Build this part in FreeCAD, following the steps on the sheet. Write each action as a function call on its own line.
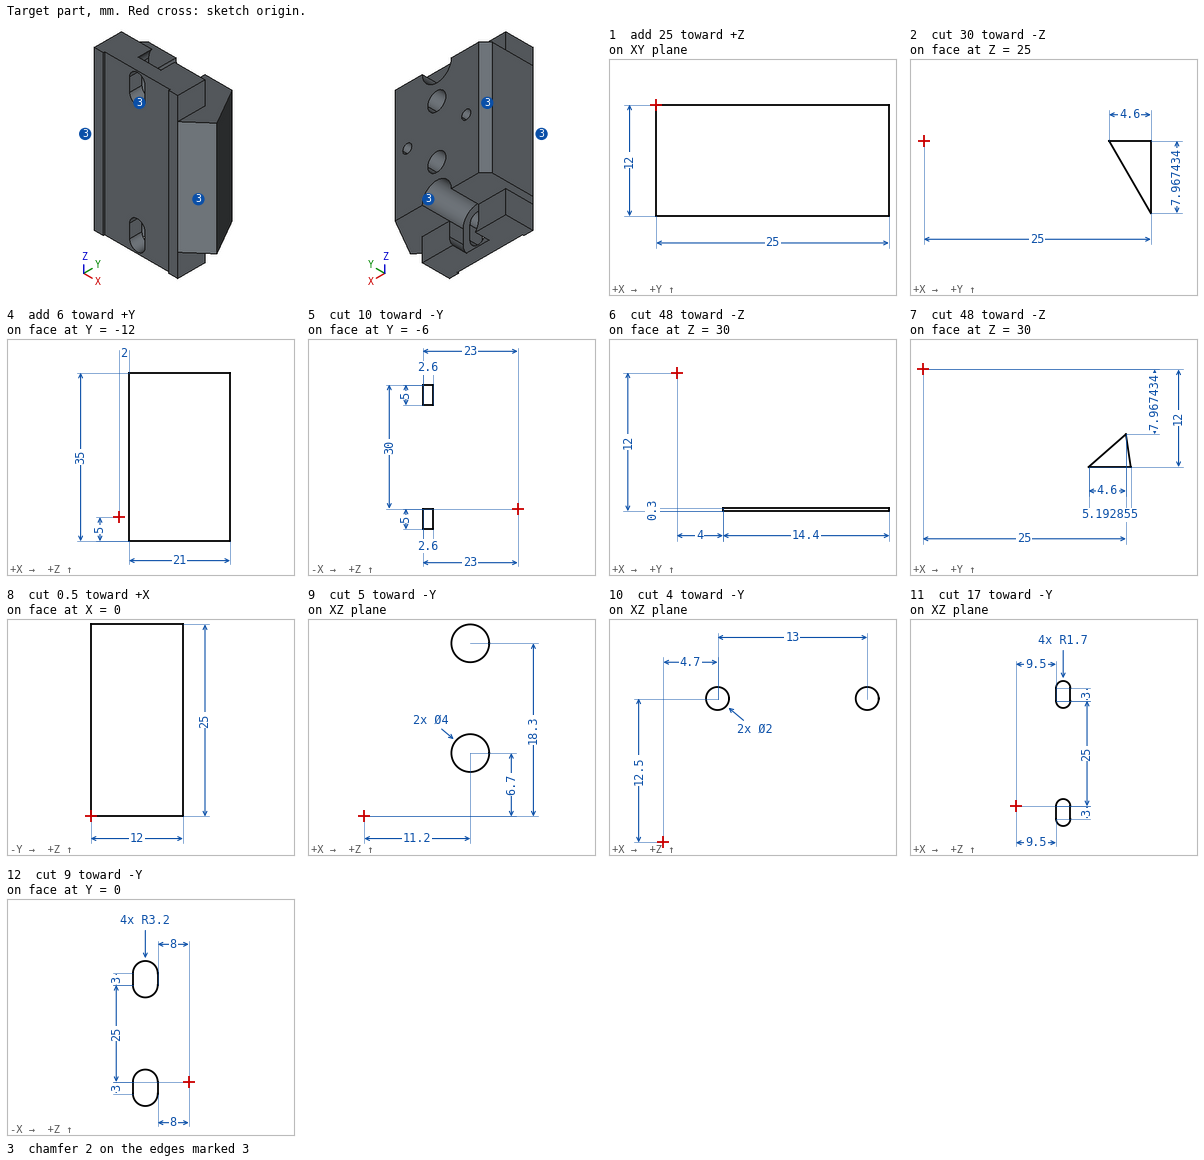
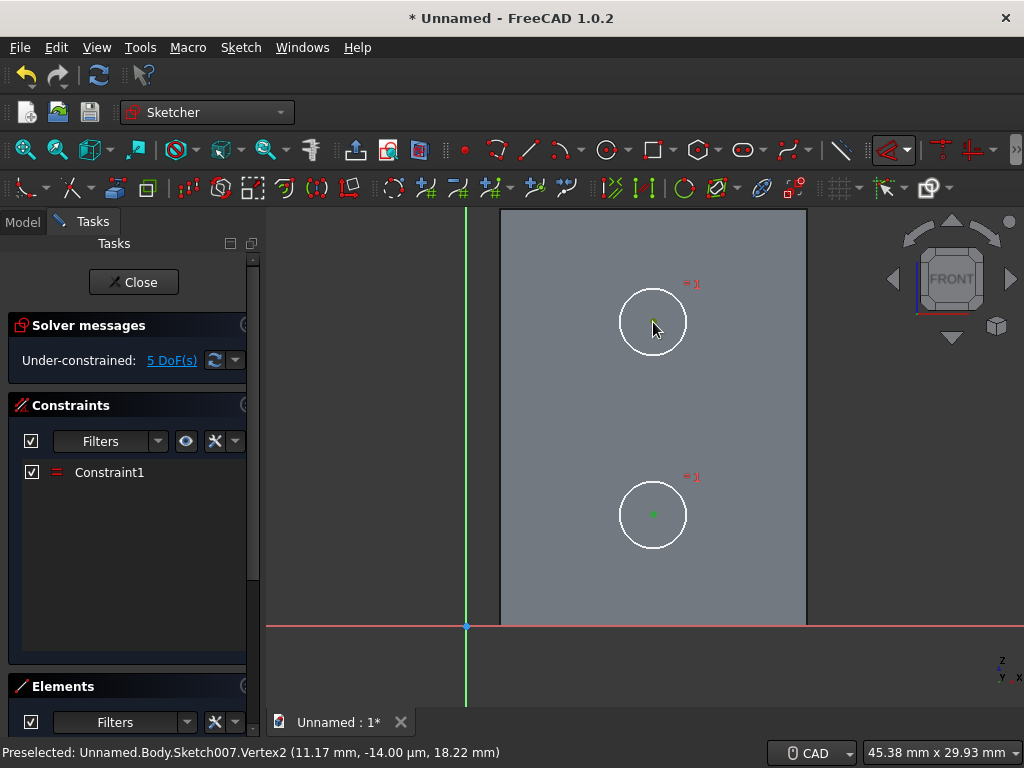
click(996, 150)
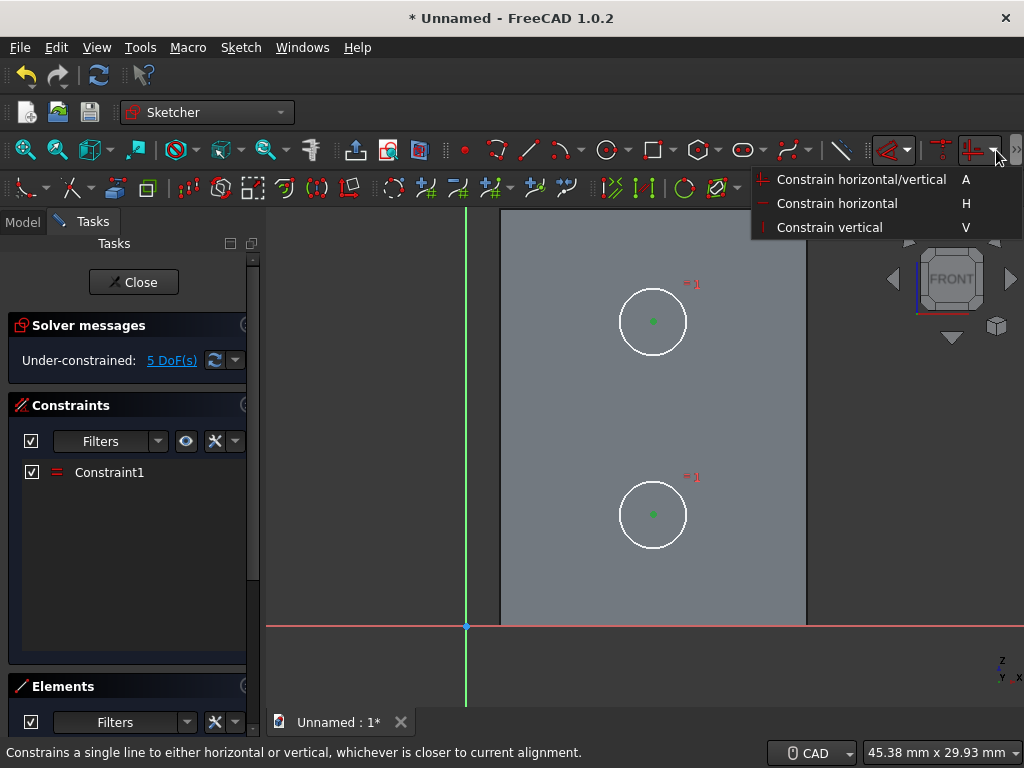
click(887, 227)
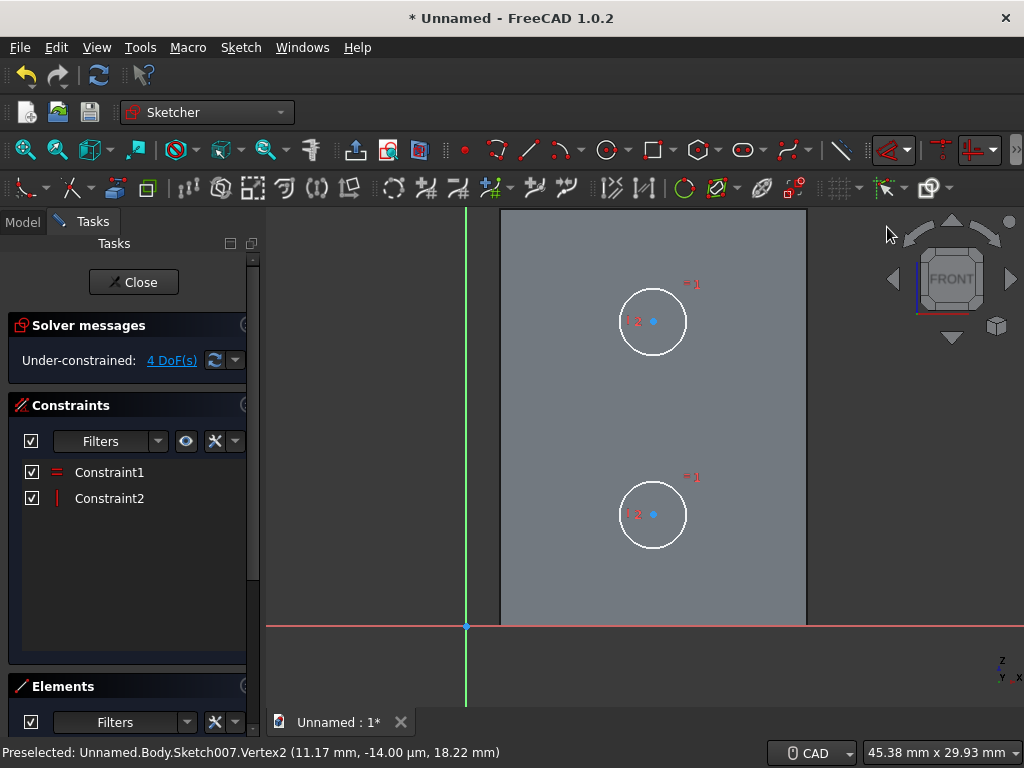
click(676, 491)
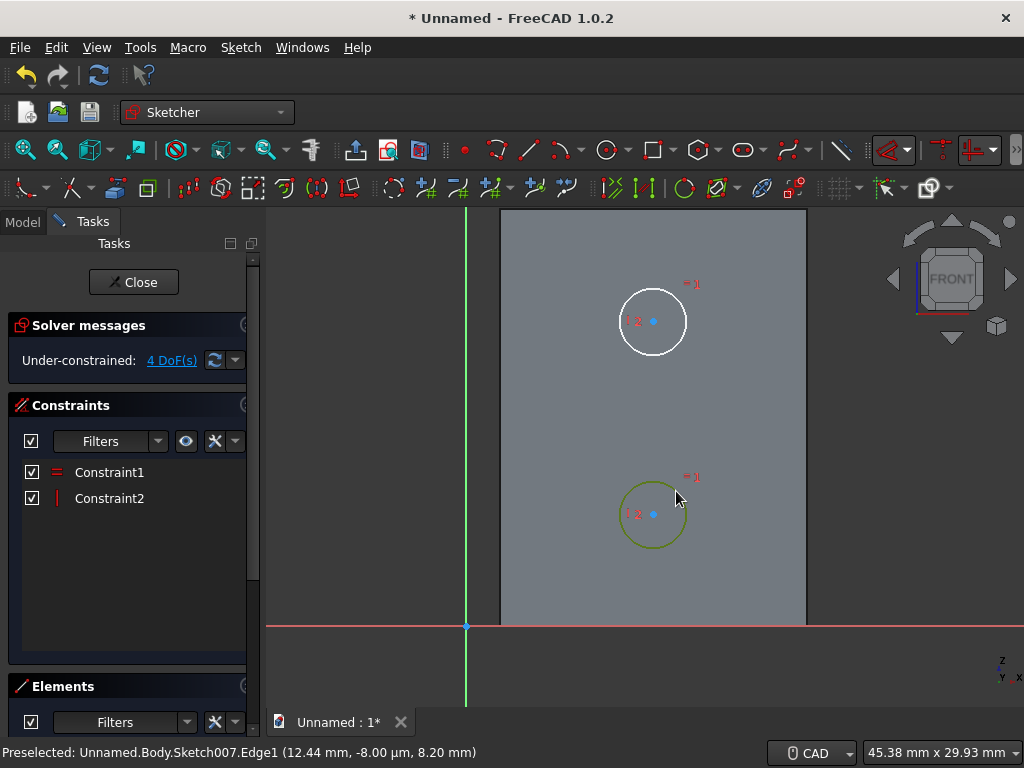
key(k)
key(o)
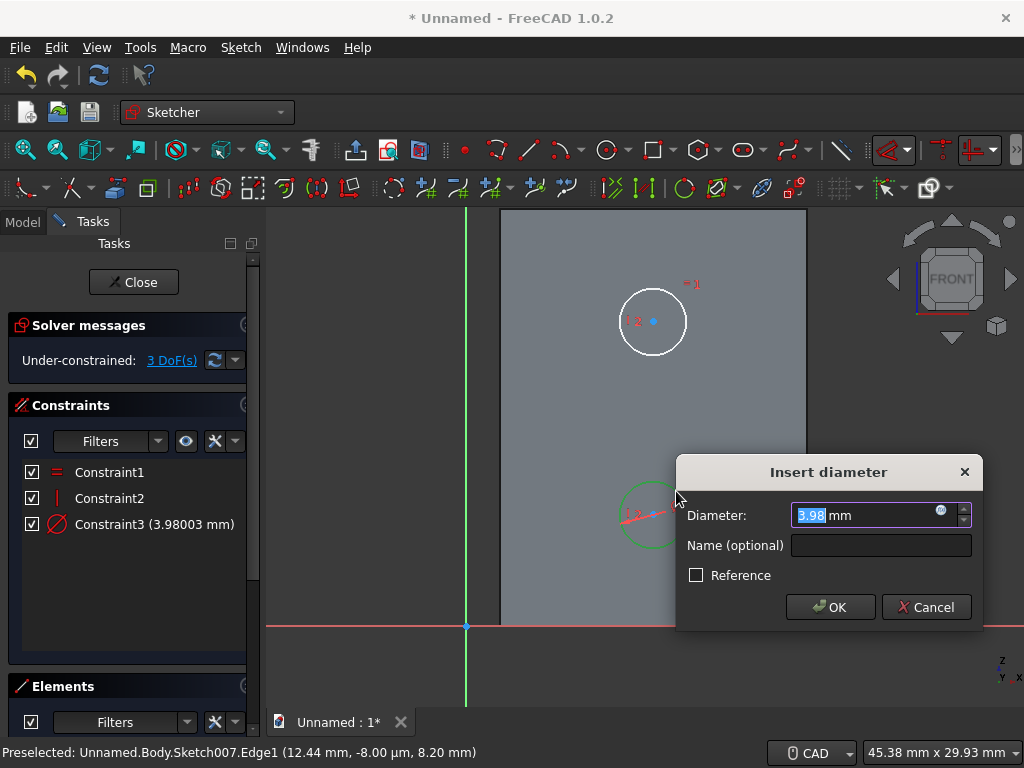
text(4)
key(Return)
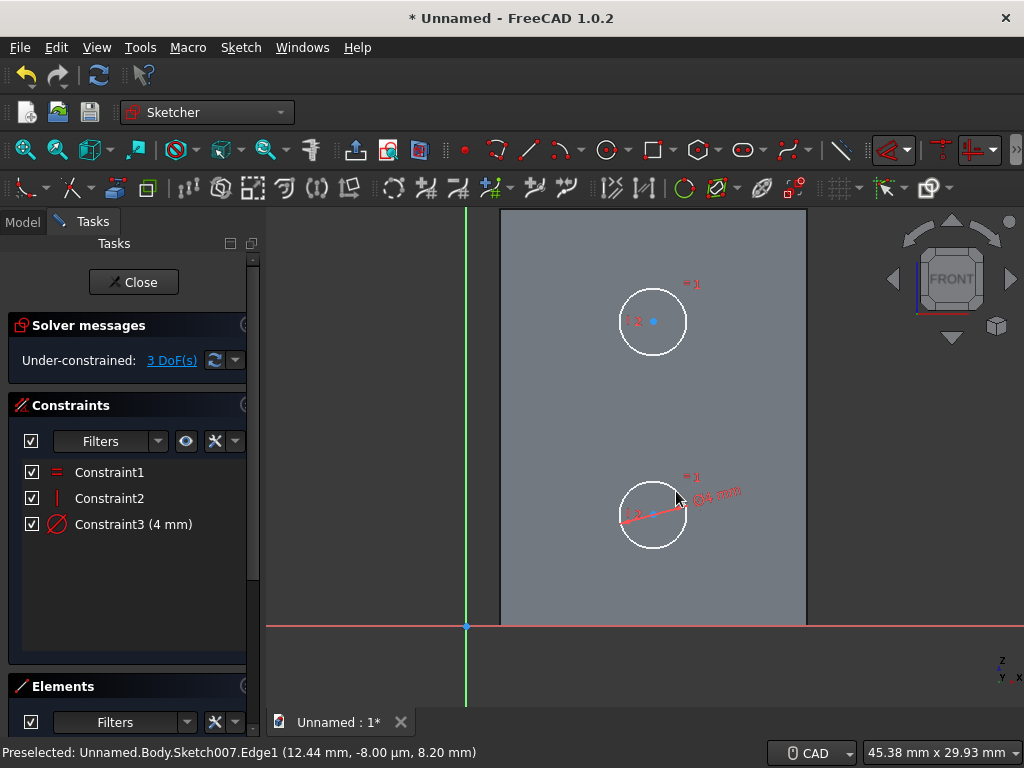
click(653, 515)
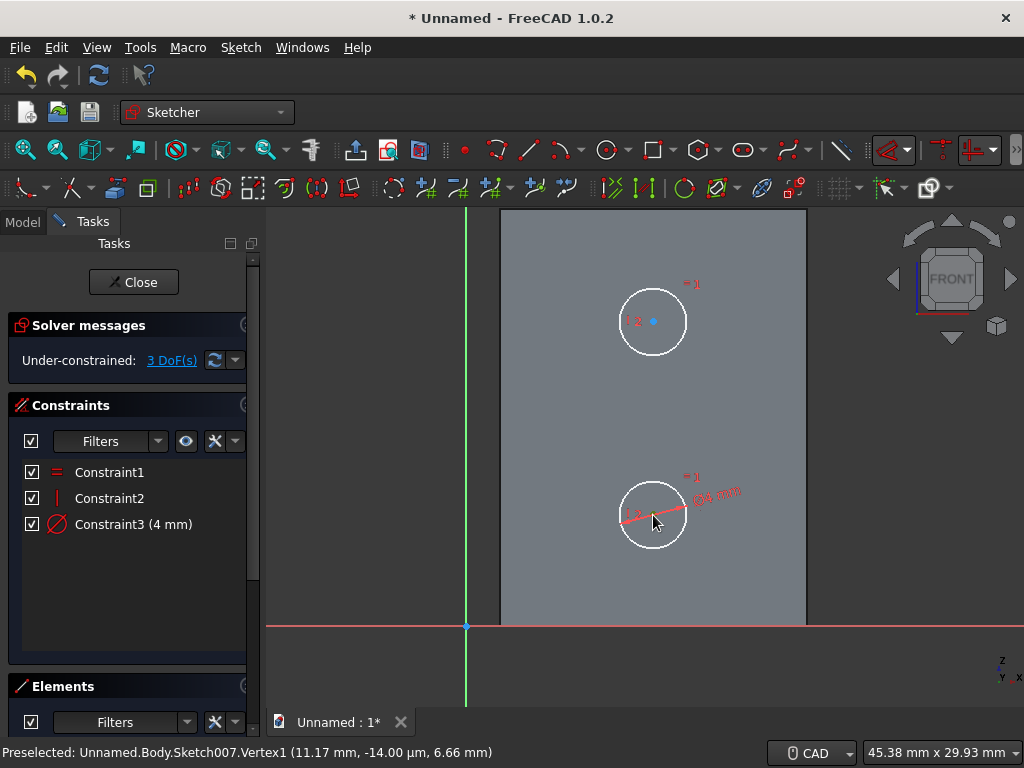
click(910, 150)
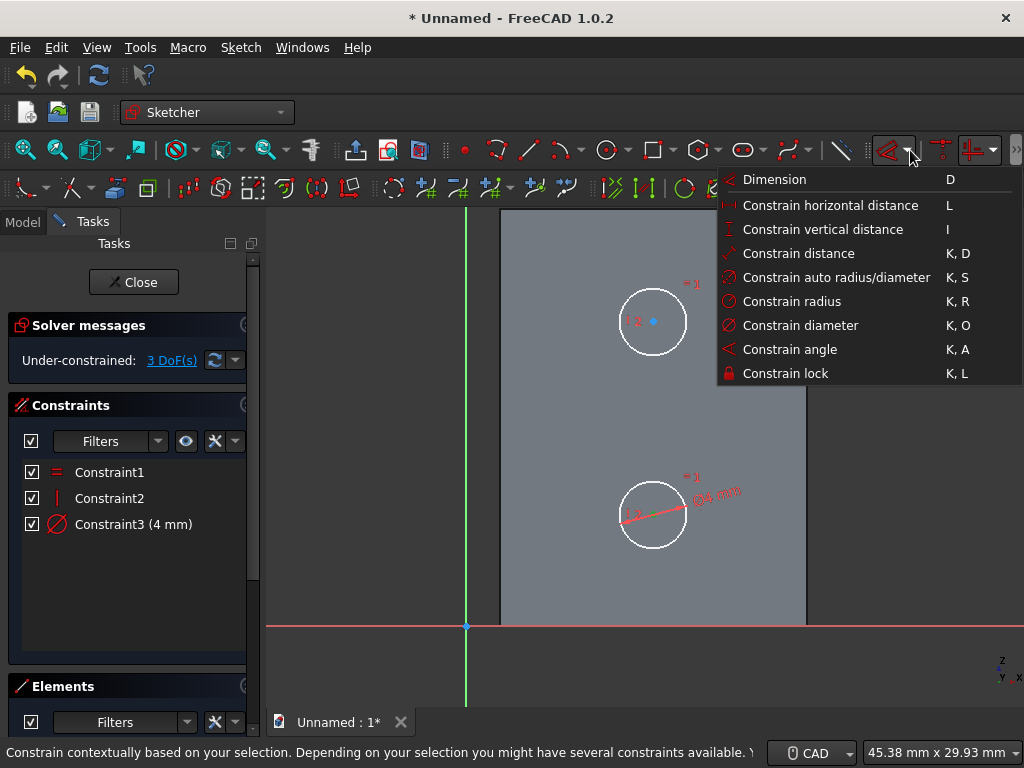
click(870, 229)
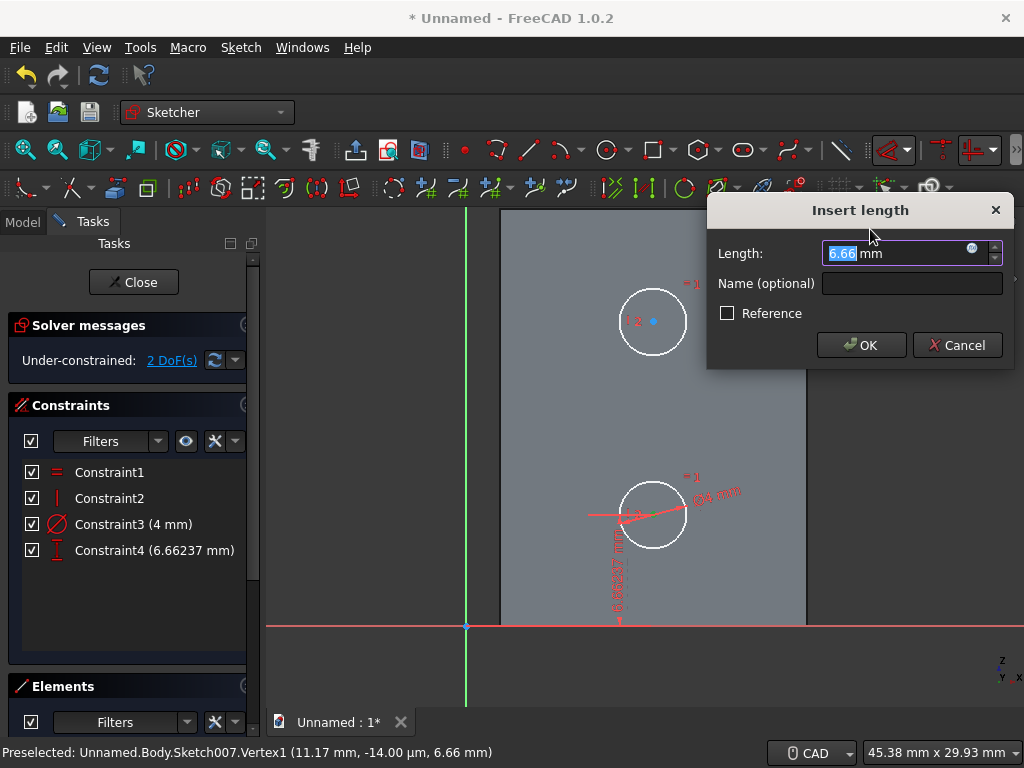
text(6.7)
key(Return)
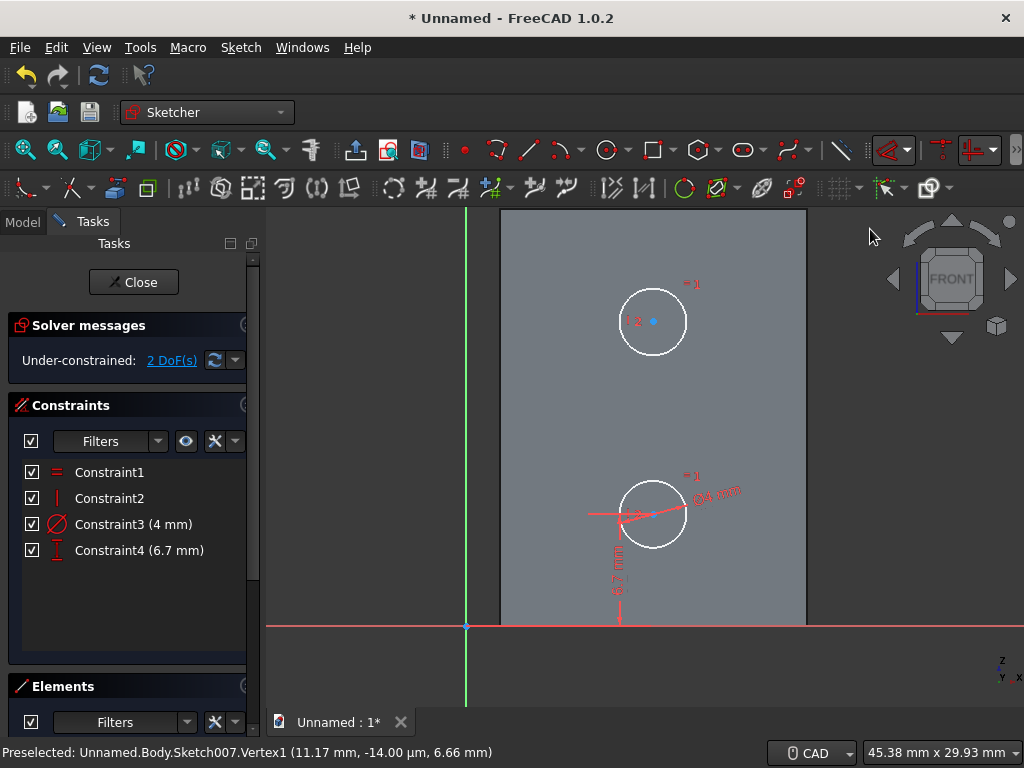
click(653, 514)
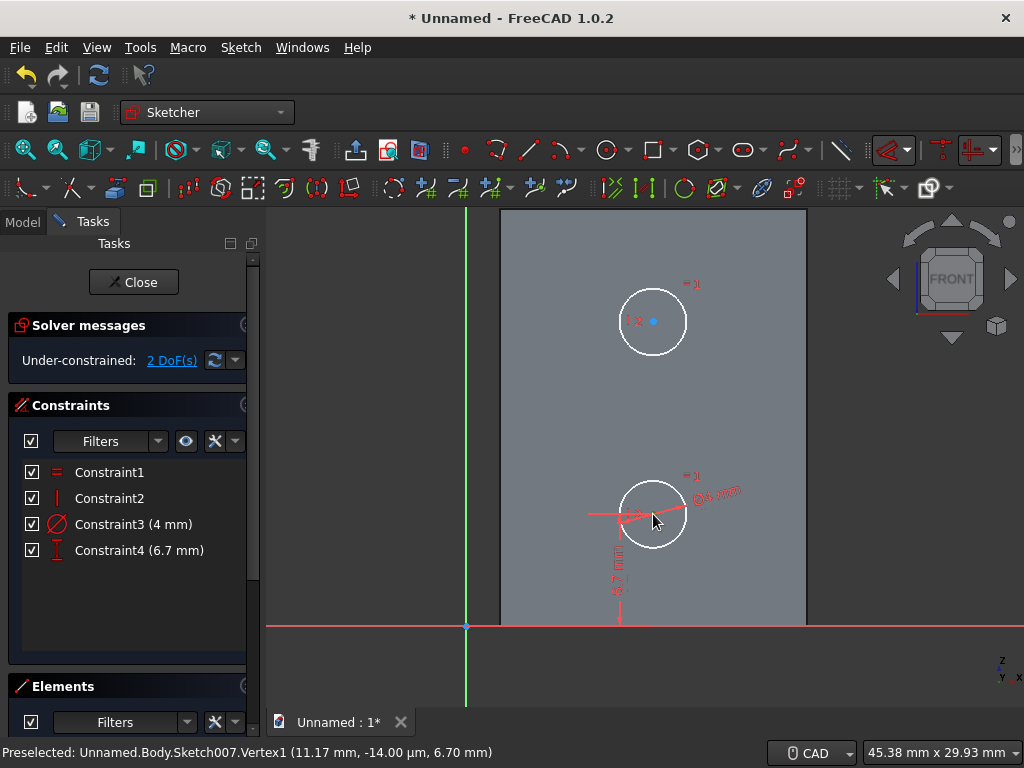
click(910, 150)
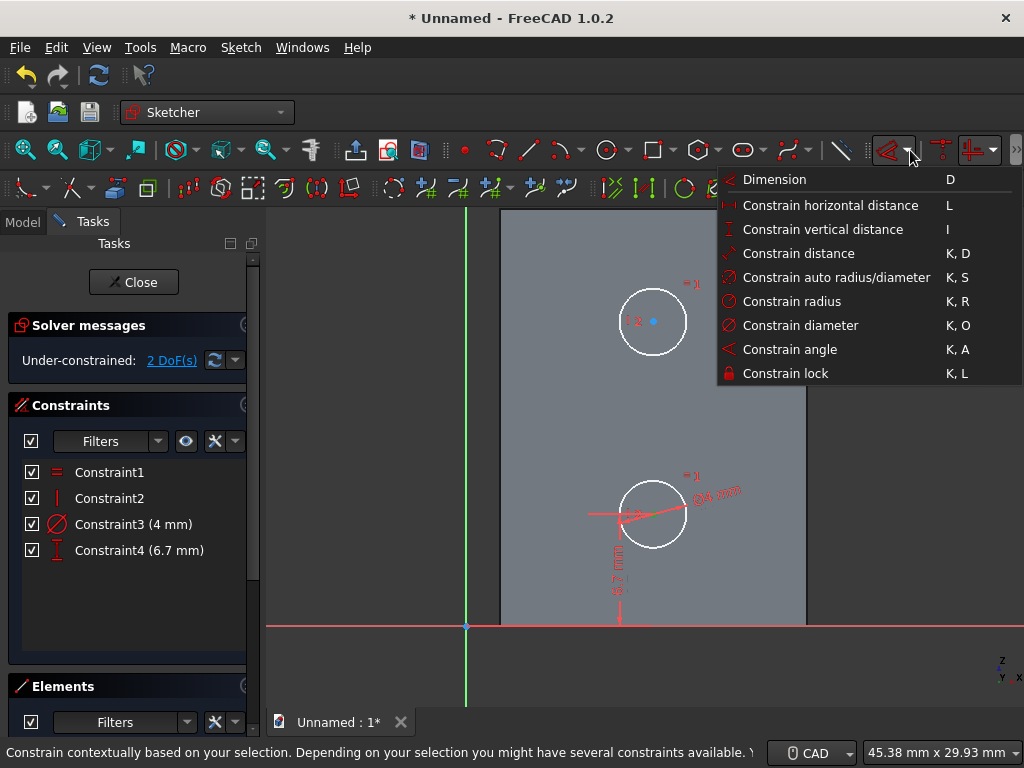
click(870, 205)